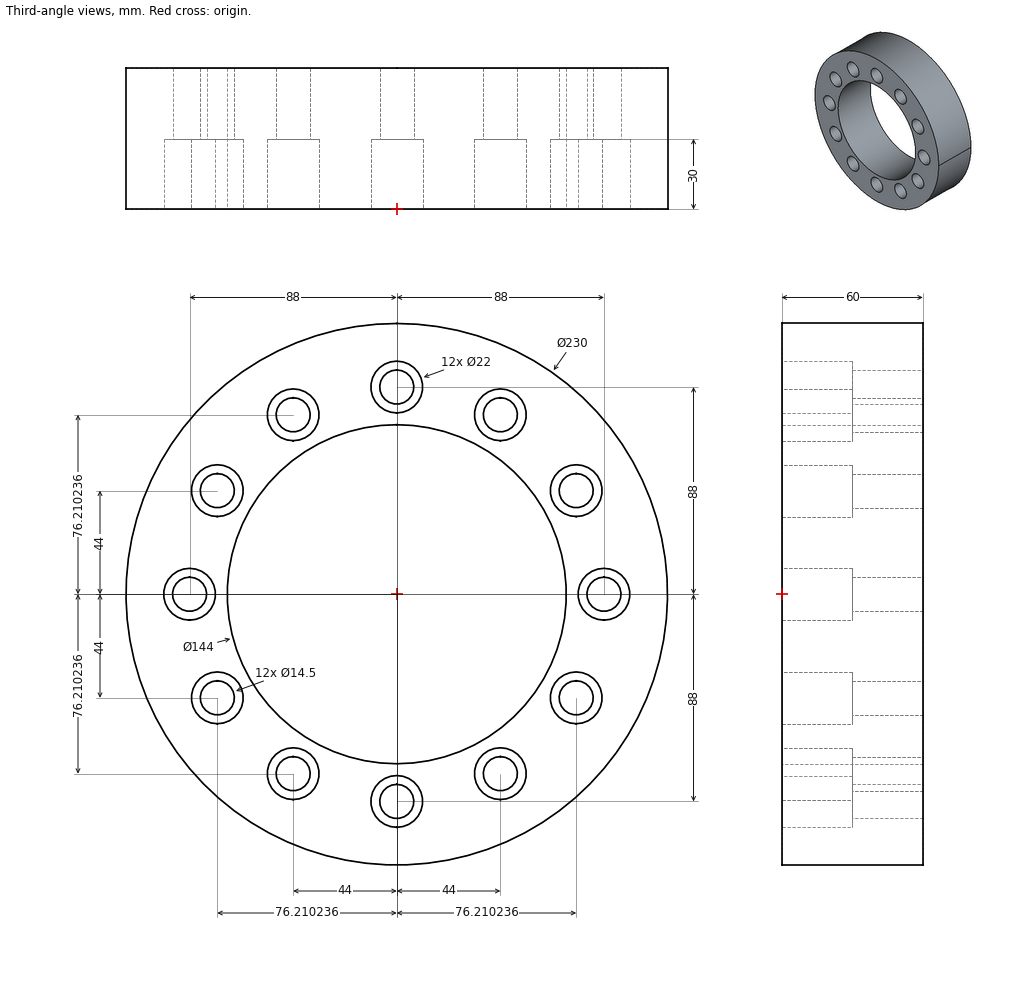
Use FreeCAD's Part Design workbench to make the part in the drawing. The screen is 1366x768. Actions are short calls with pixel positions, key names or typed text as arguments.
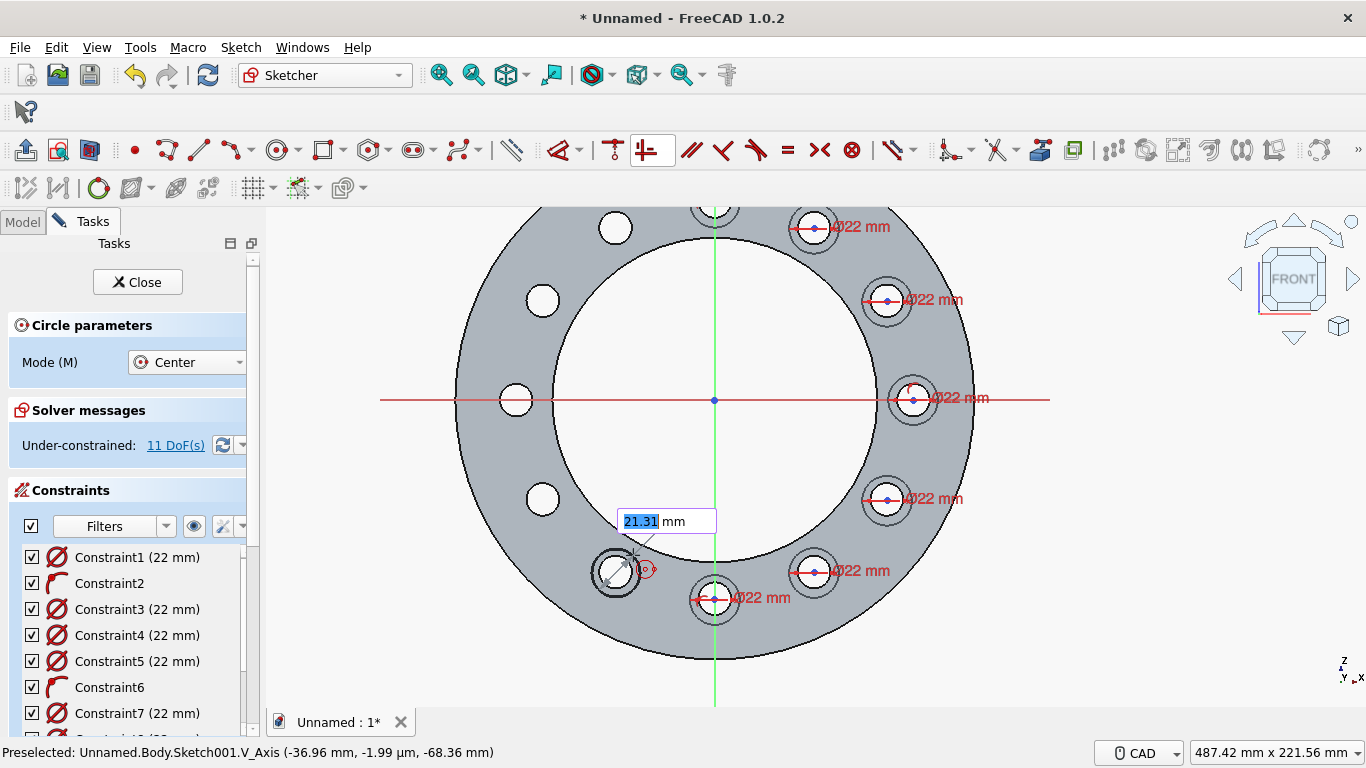
text(22)
key(Return)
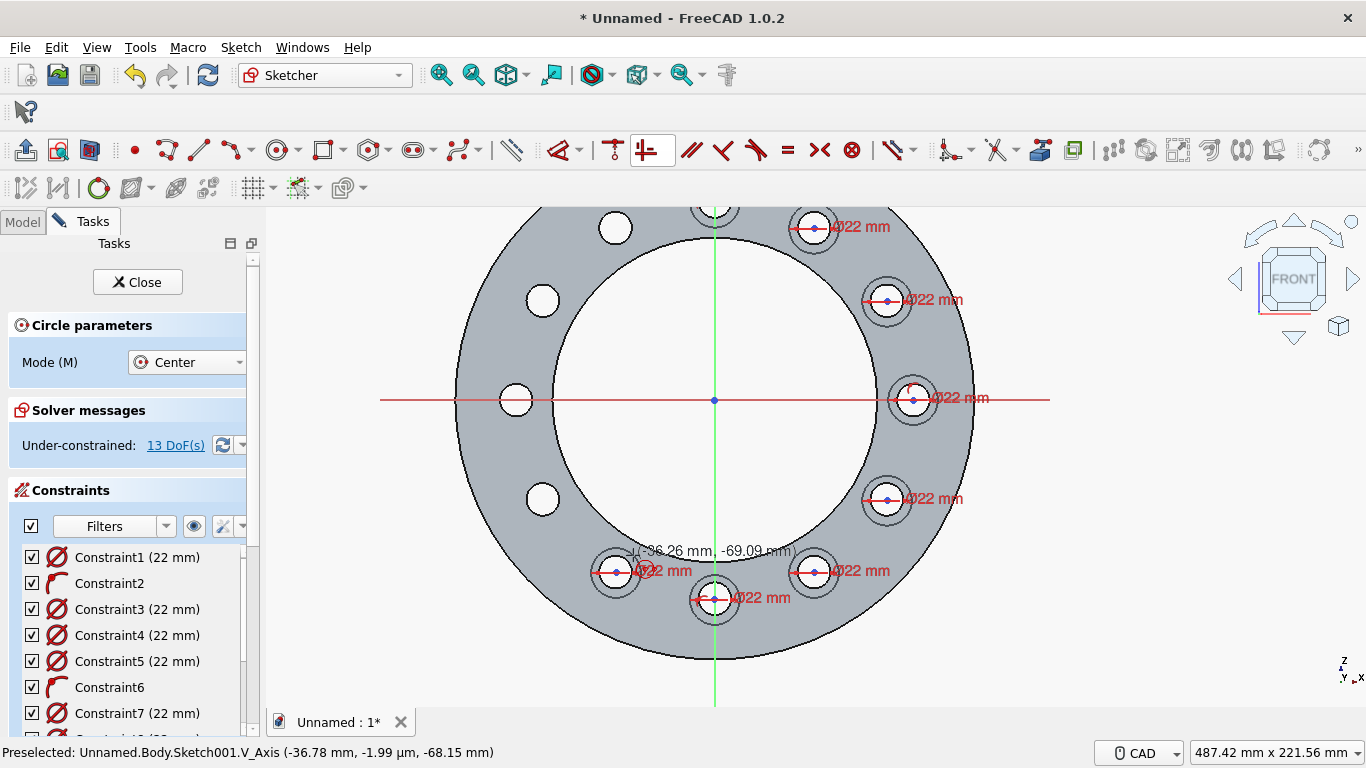
click(543, 499)
move(560, 482)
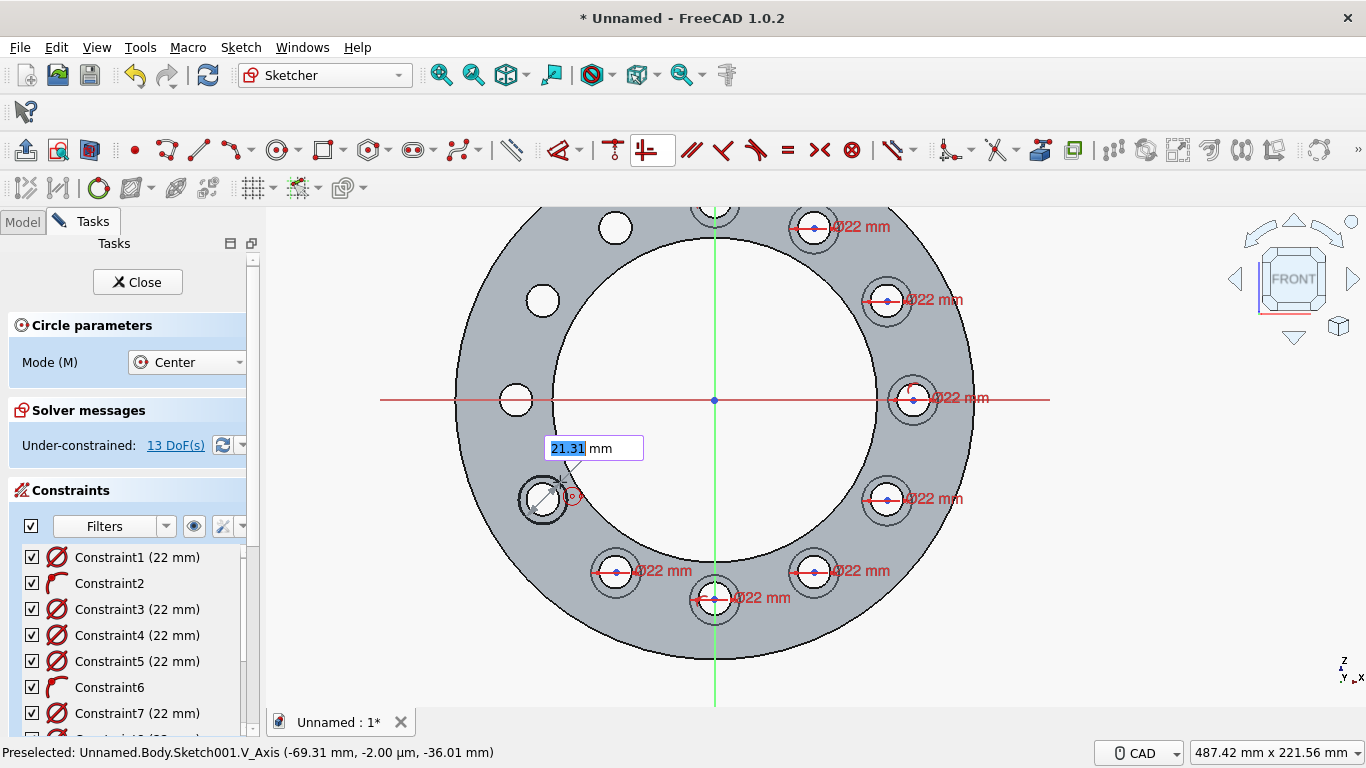
text(22)
key(Return)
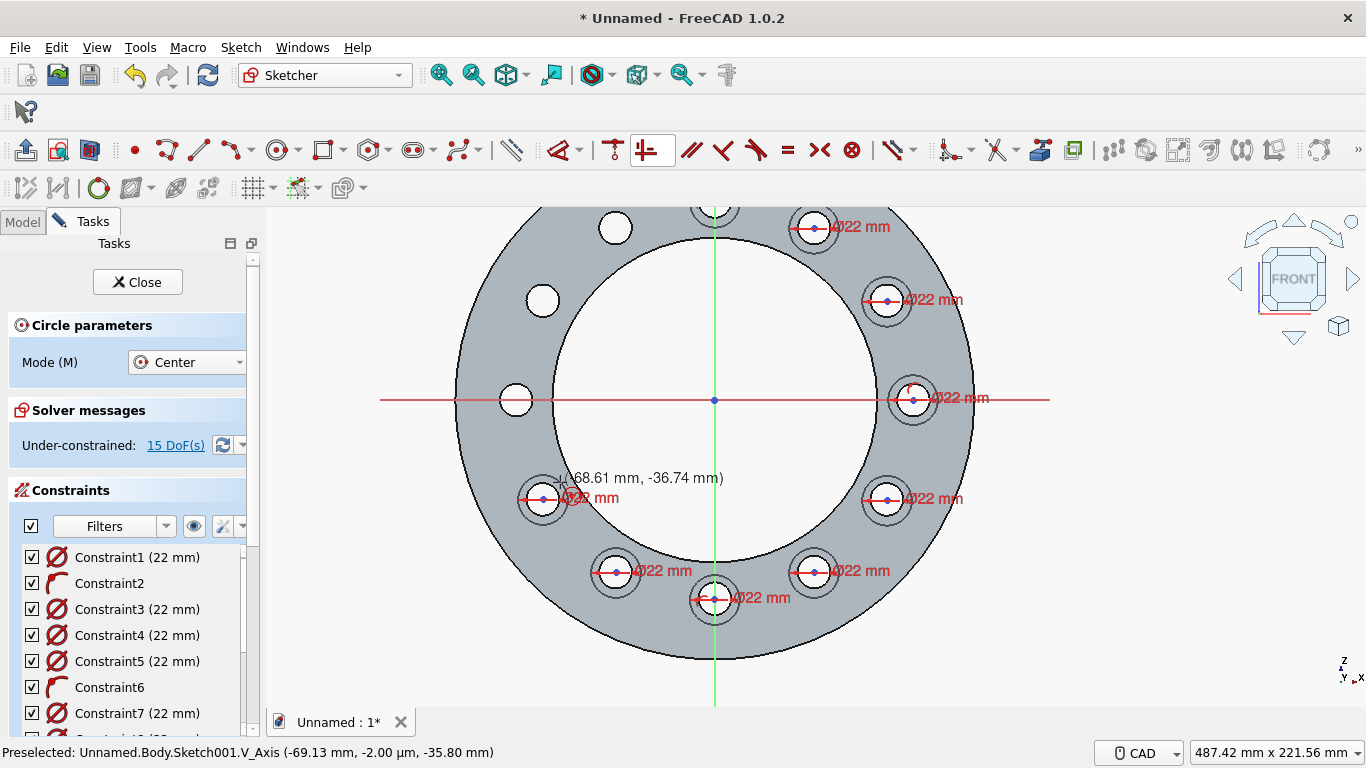
click(516, 400)
move(534, 383)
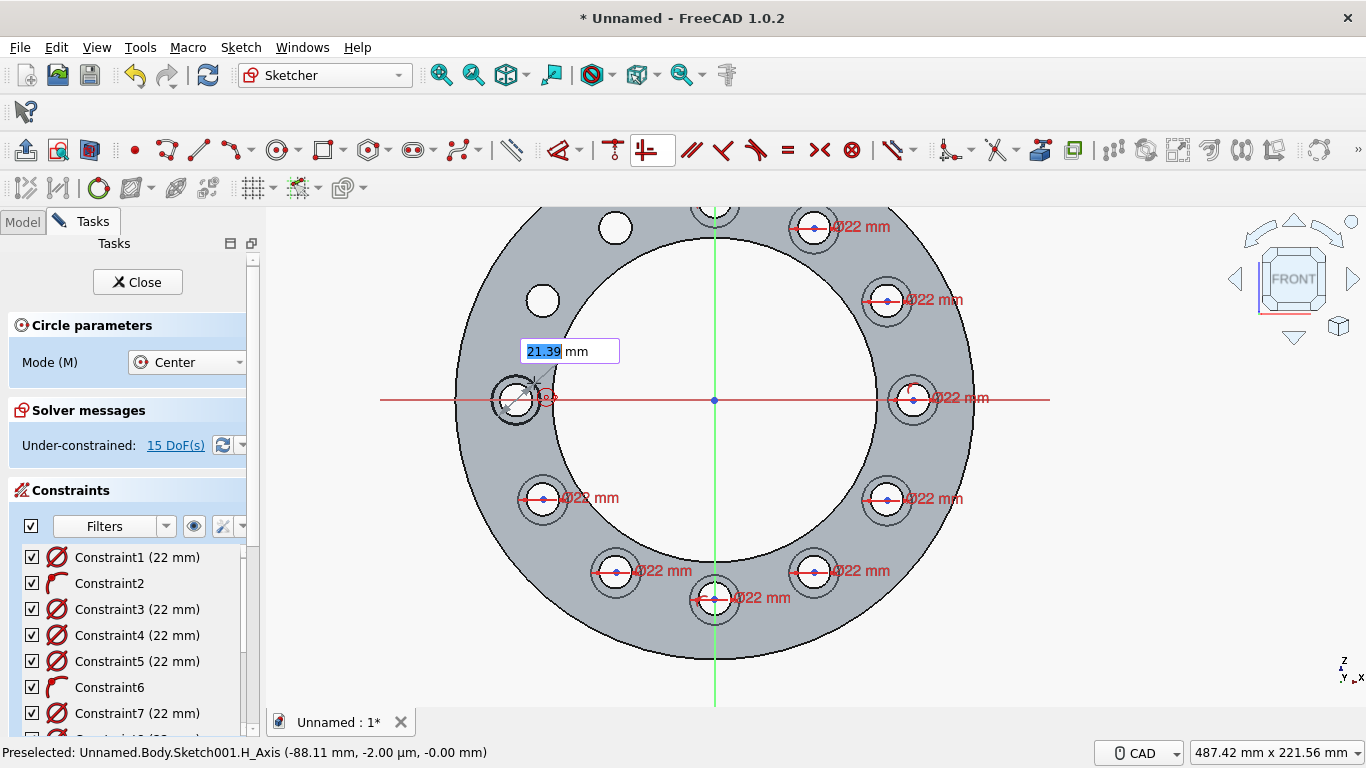
text(22)
key(Return)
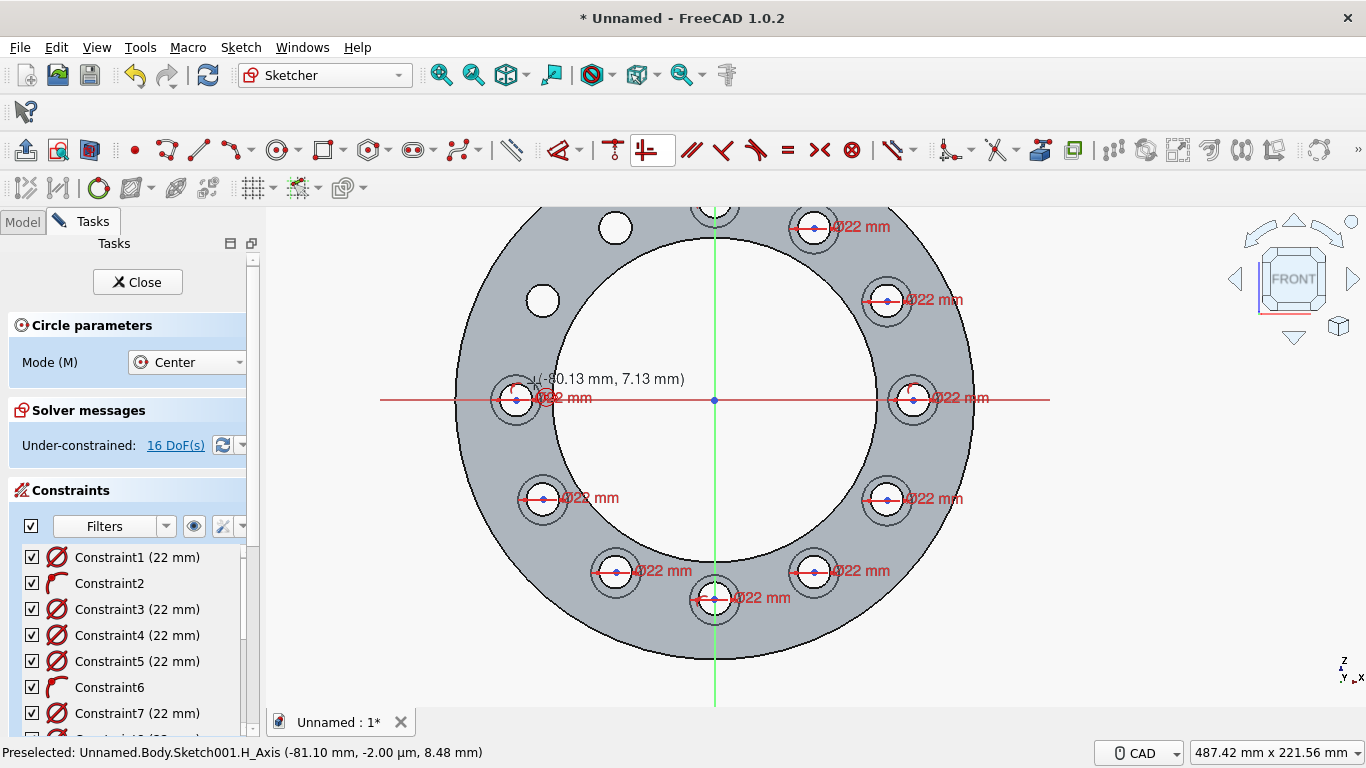
click(543, 301)
move(560, 283)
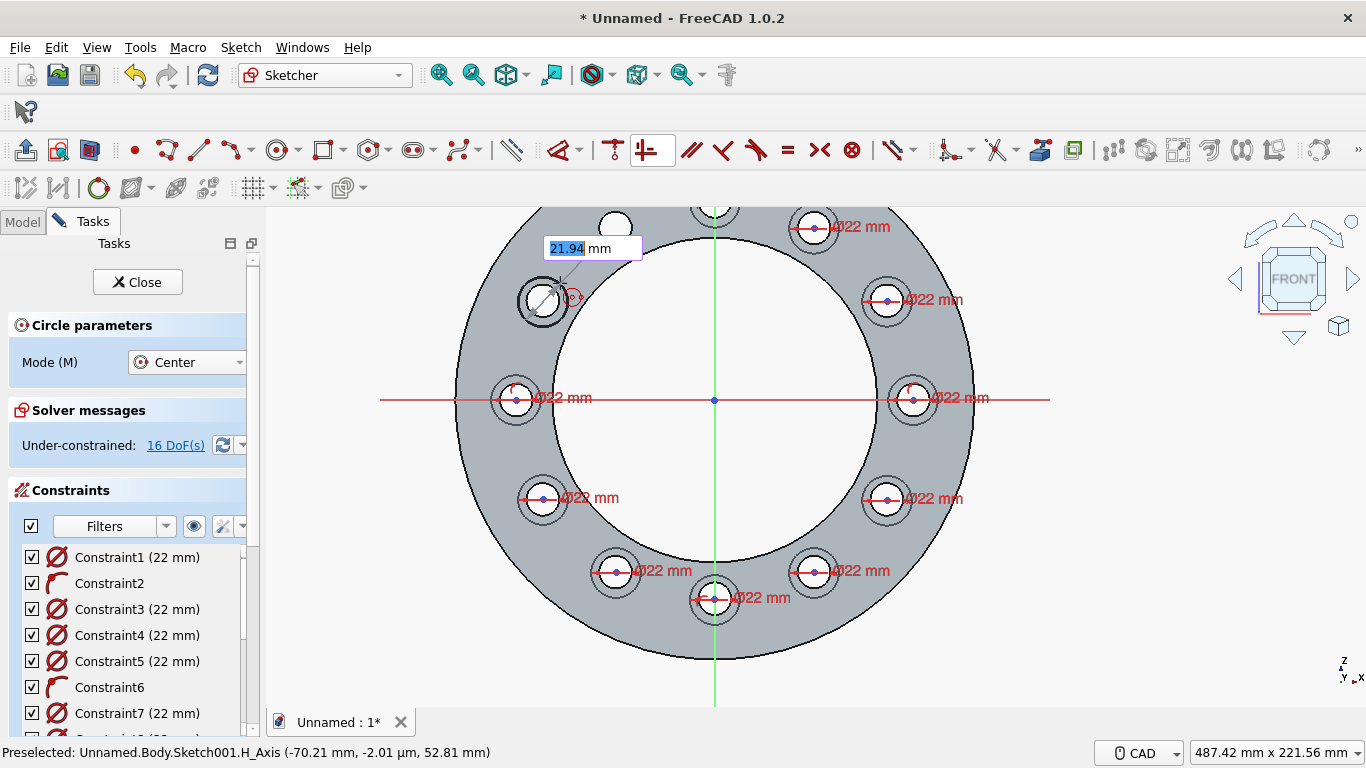
text(22)
key(Return)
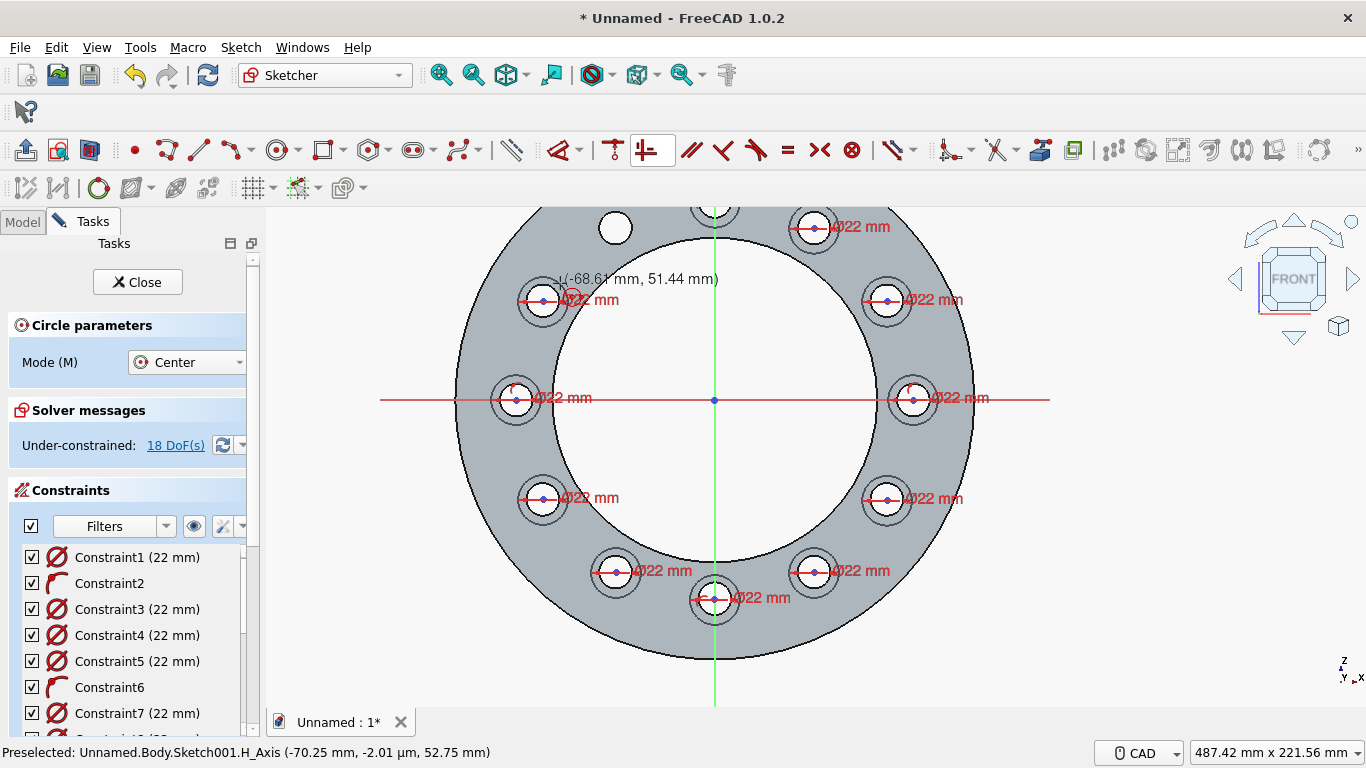
scroll(814, 573, down, 2)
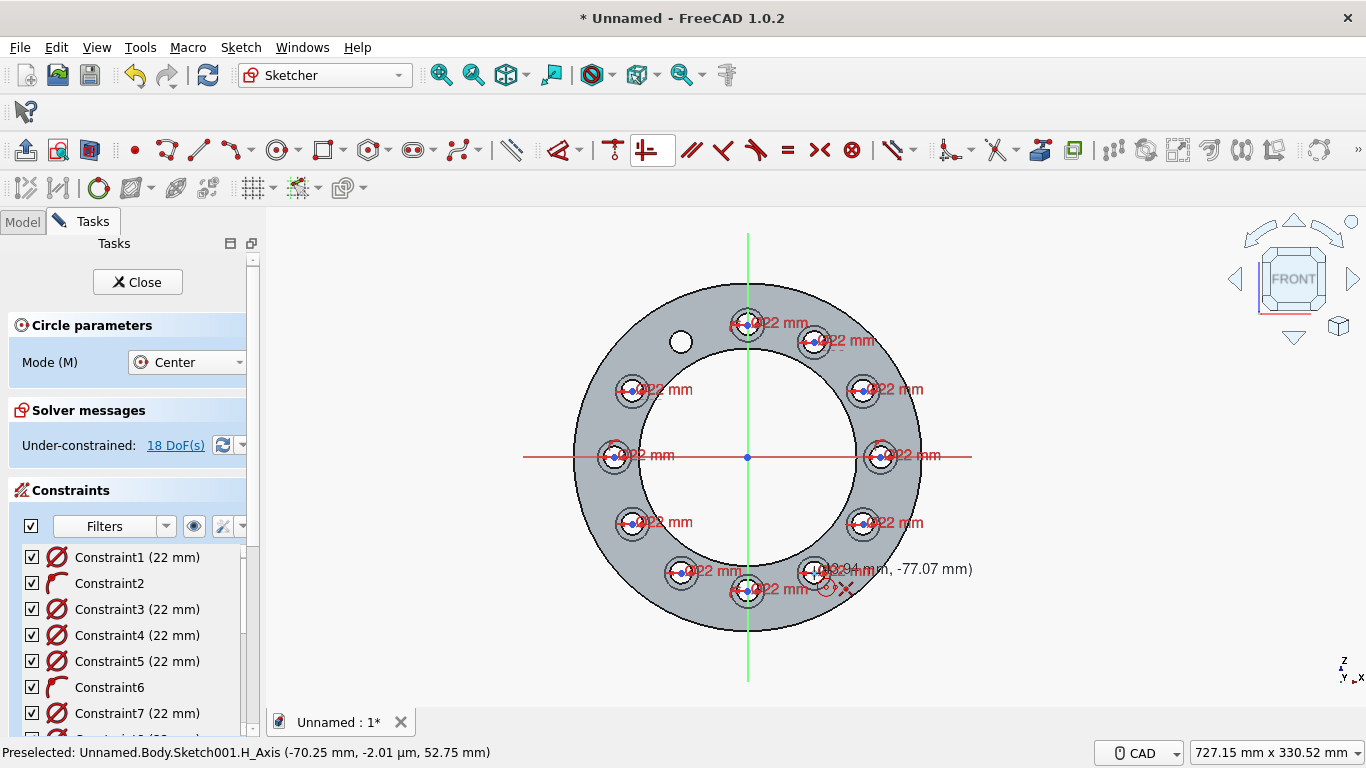
scroll(681, 342, up, 2)